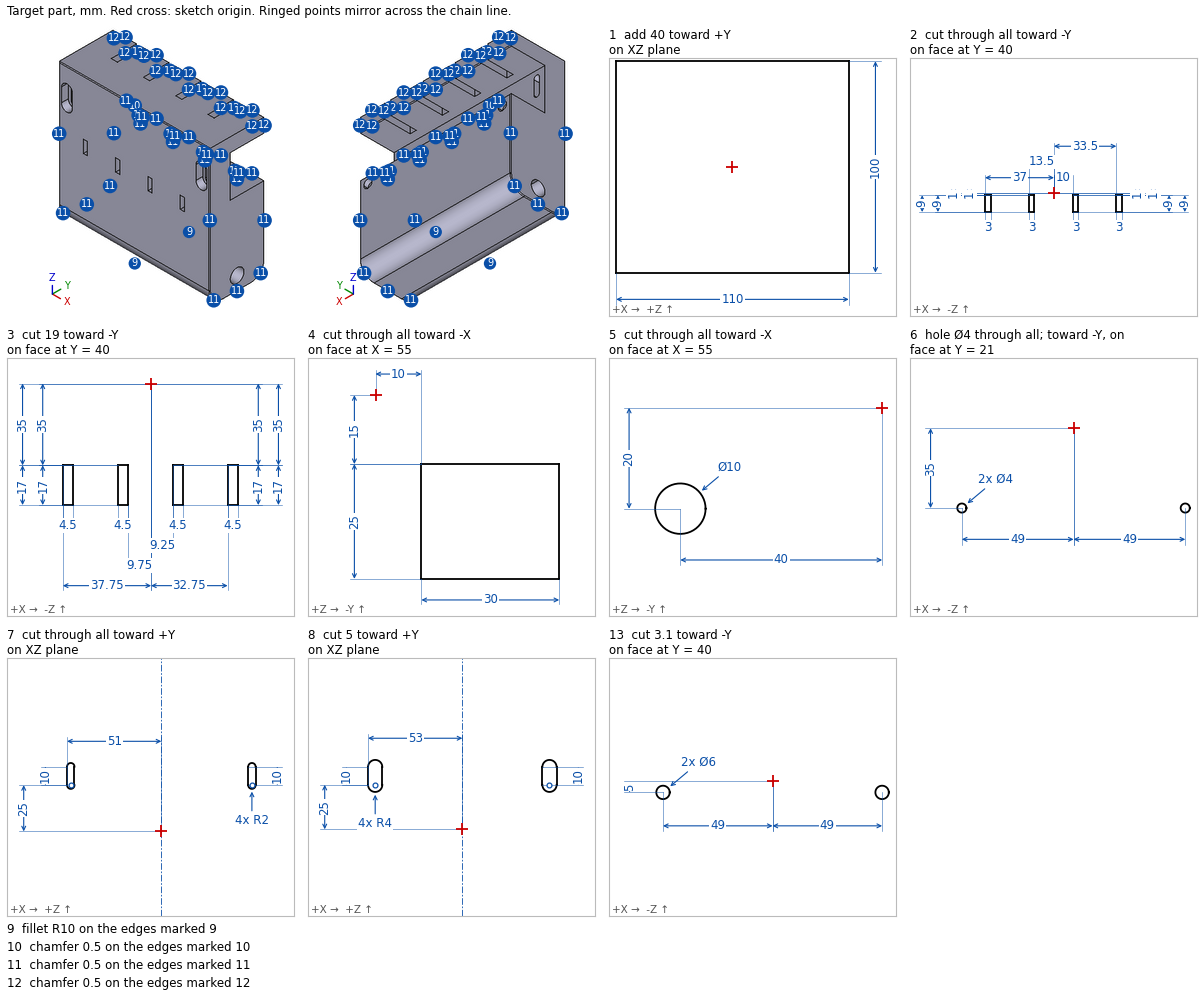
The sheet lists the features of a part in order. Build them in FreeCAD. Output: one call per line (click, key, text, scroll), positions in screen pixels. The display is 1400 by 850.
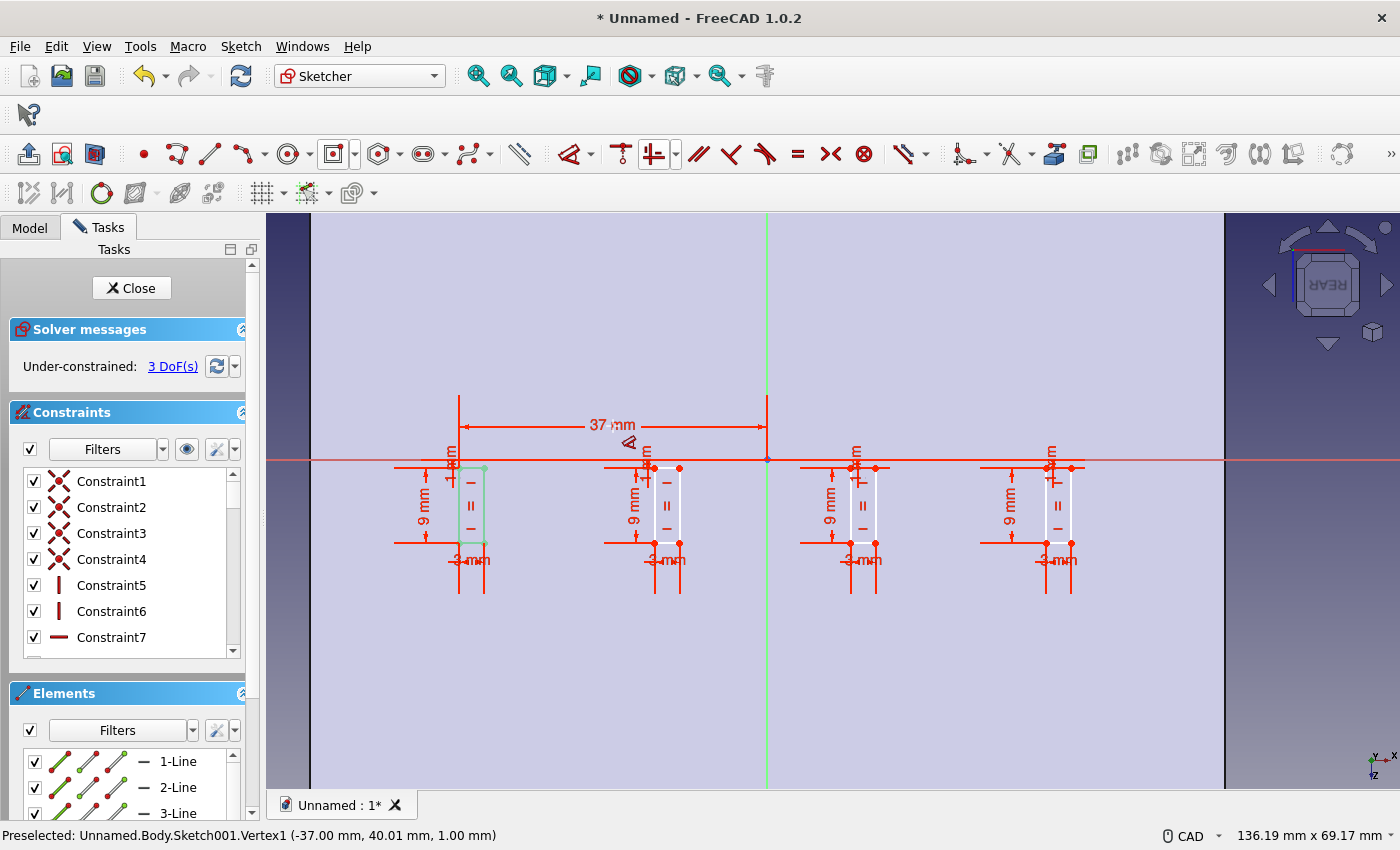
click(851, 468)
click(809, 426)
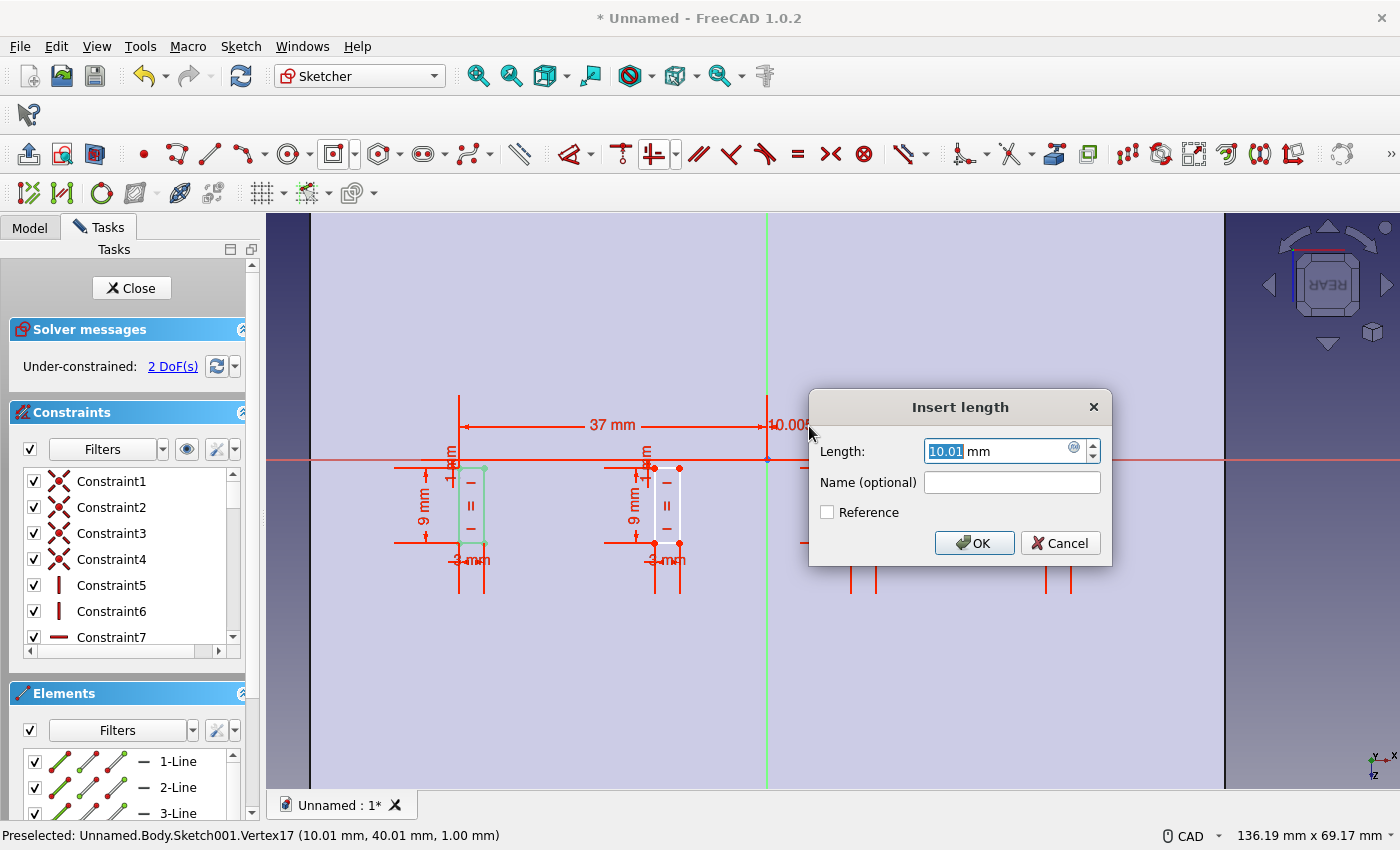
text(10)
key(Return)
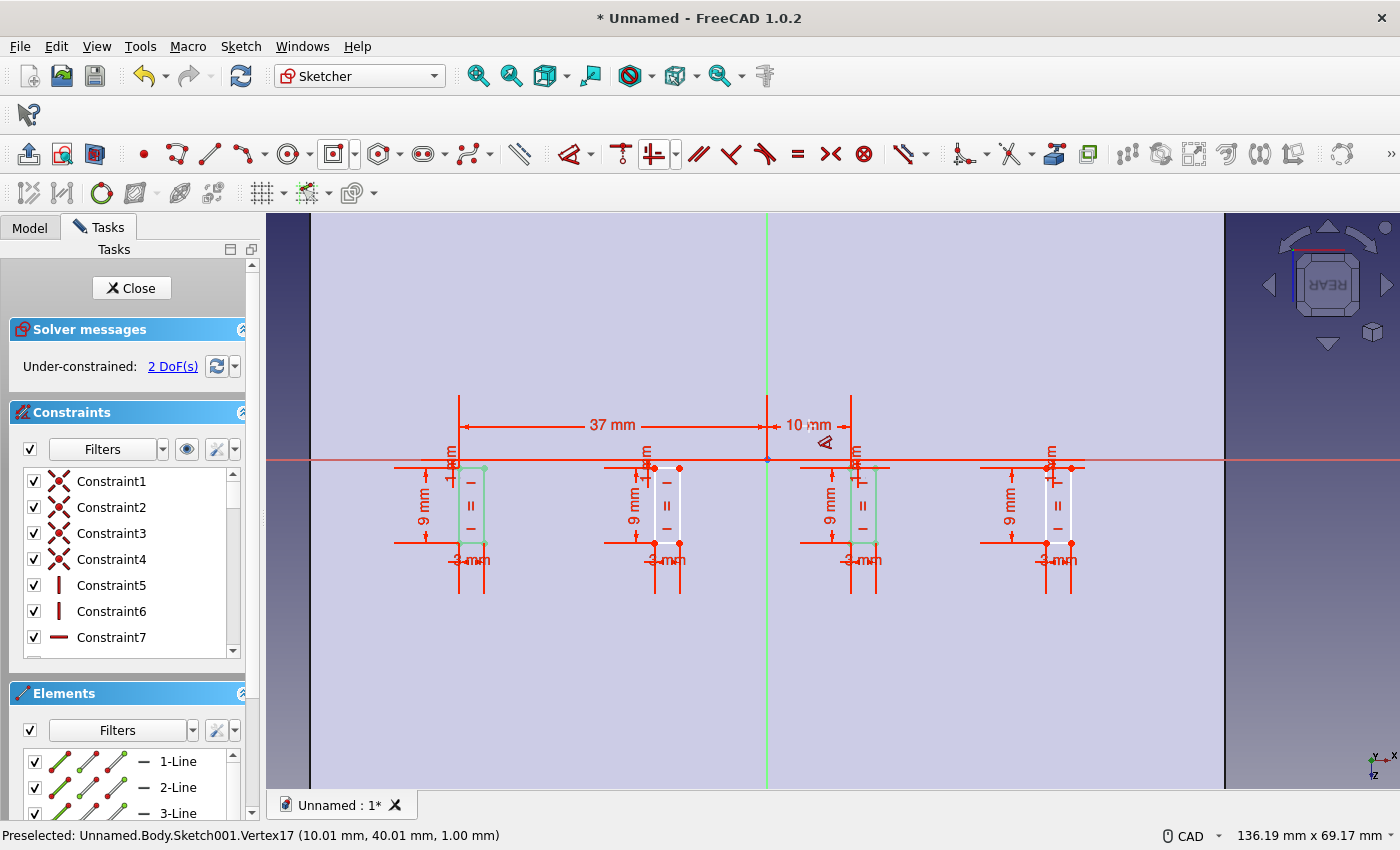
click(655, 468)
click(711, 426)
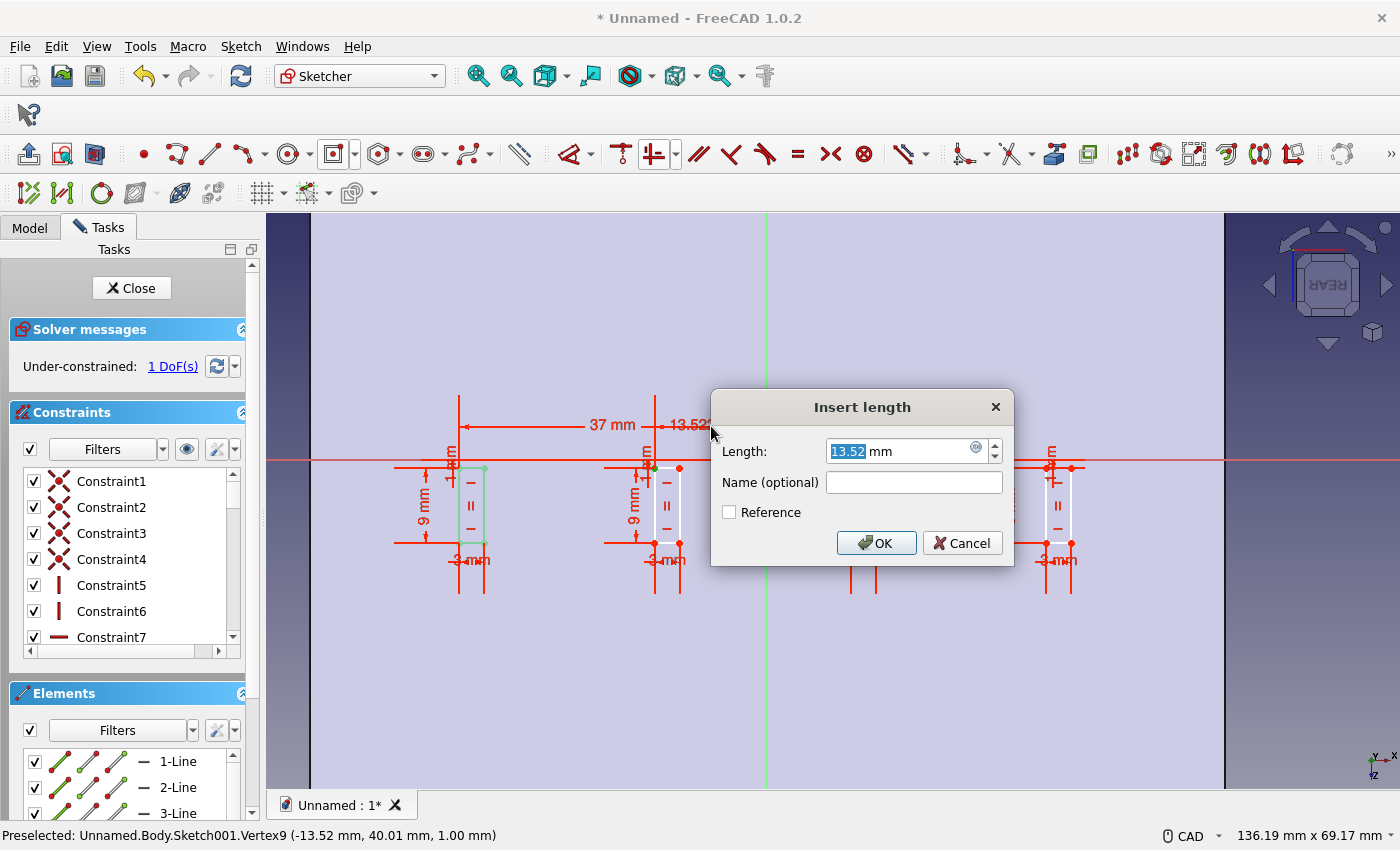
text(13.5)
key(Return)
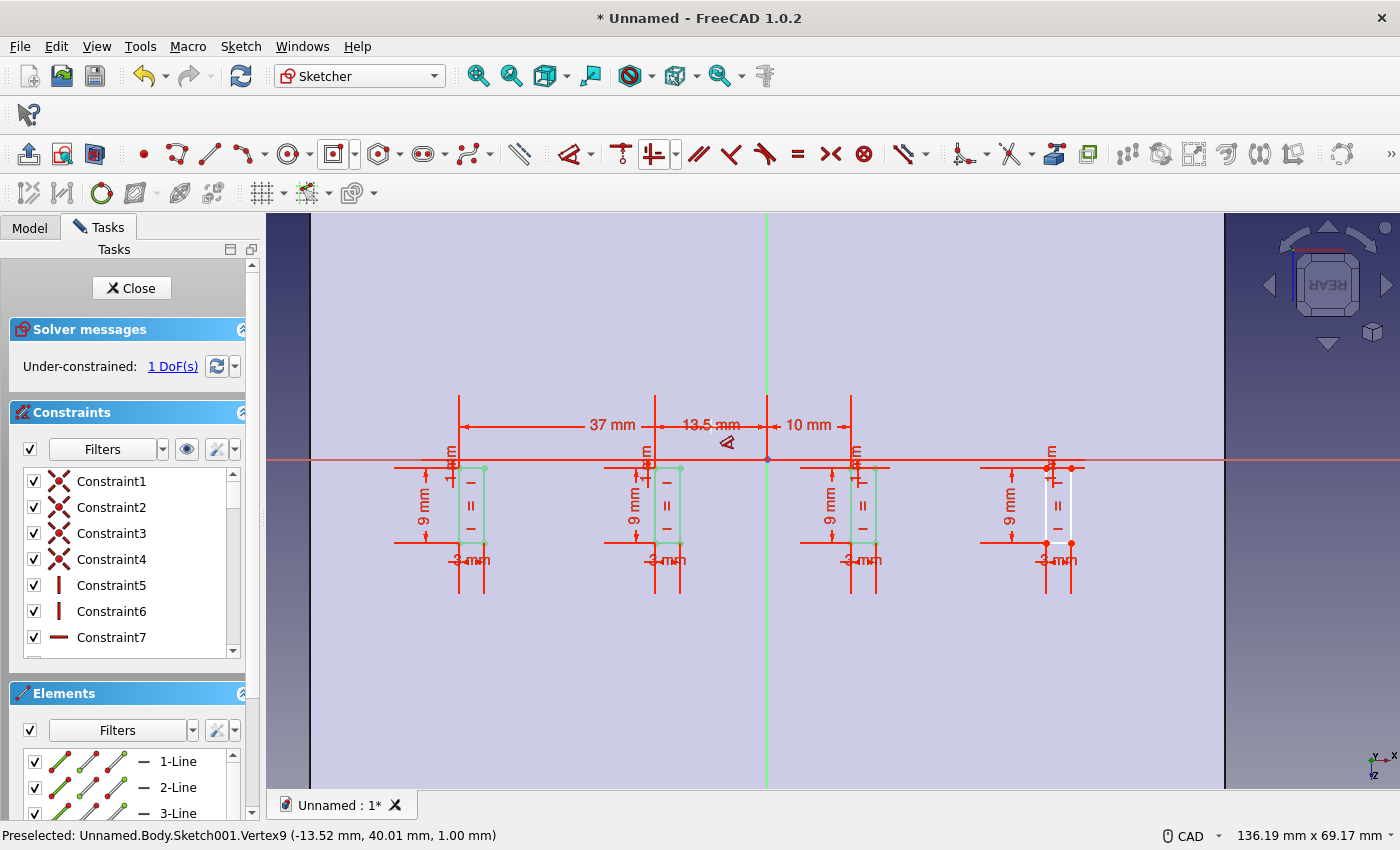
click(1046, 468)
click(907, 426)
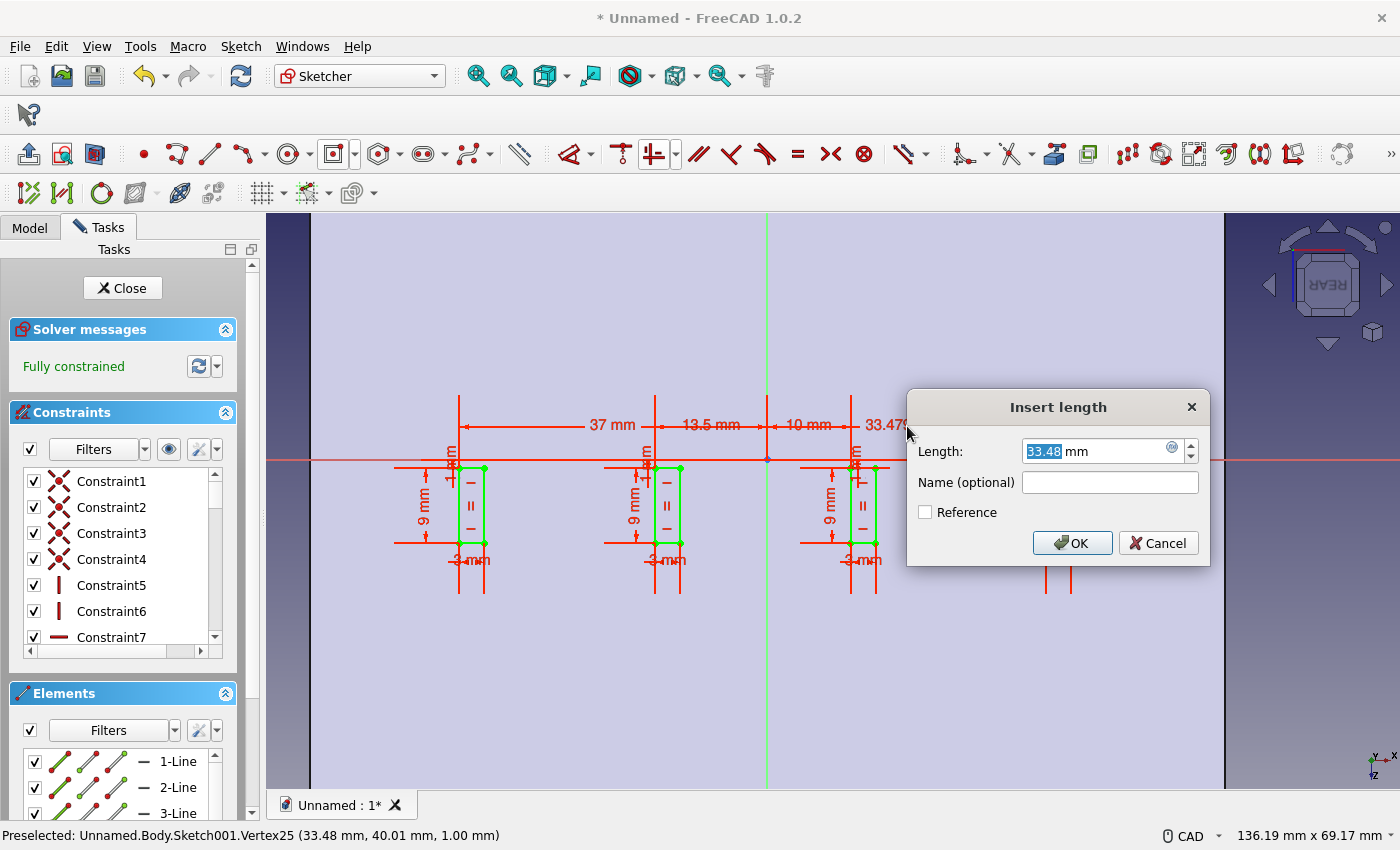
text(33.5)
key(Return)
key(Escape)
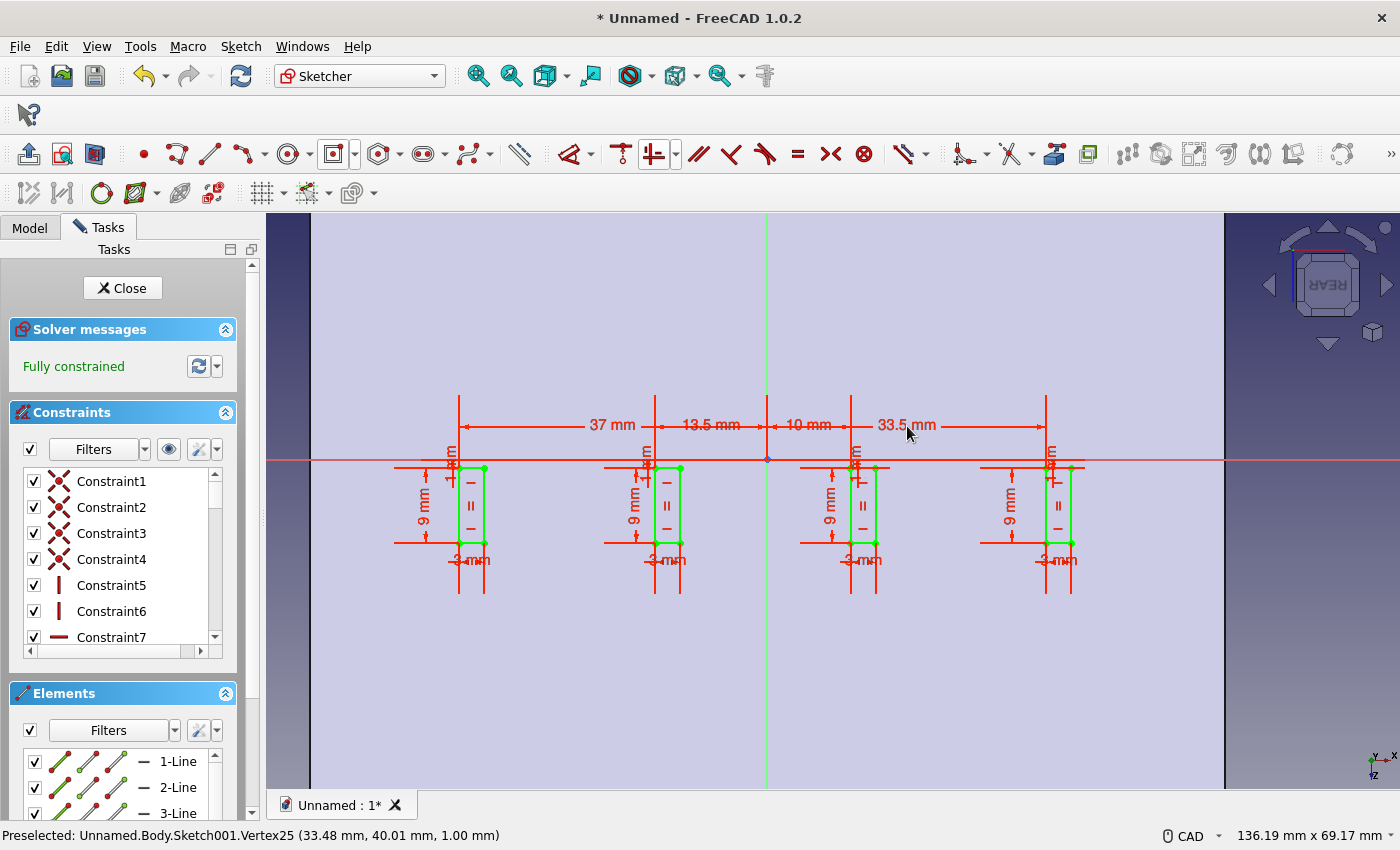
click(123, 288)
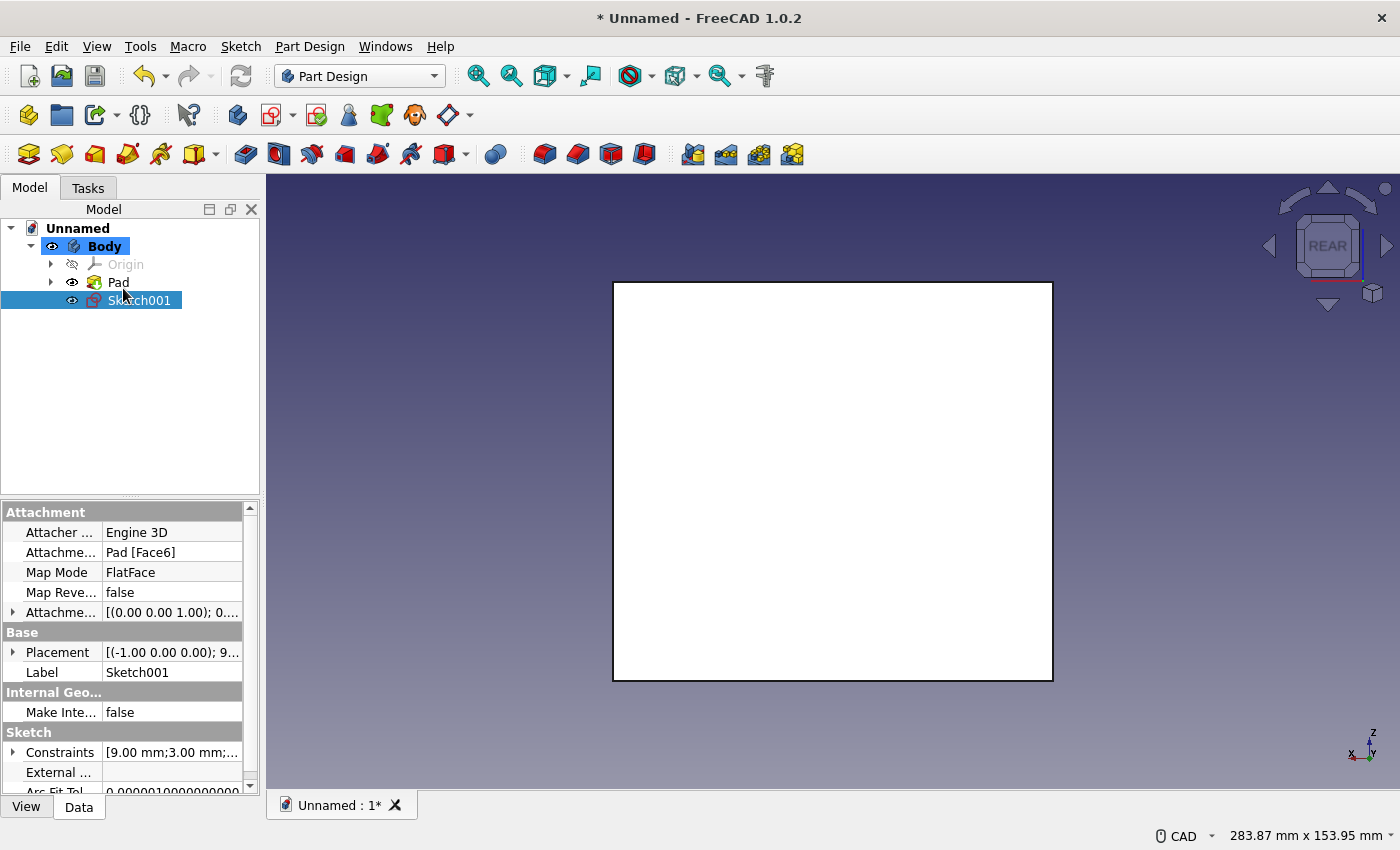
click(246, 154)